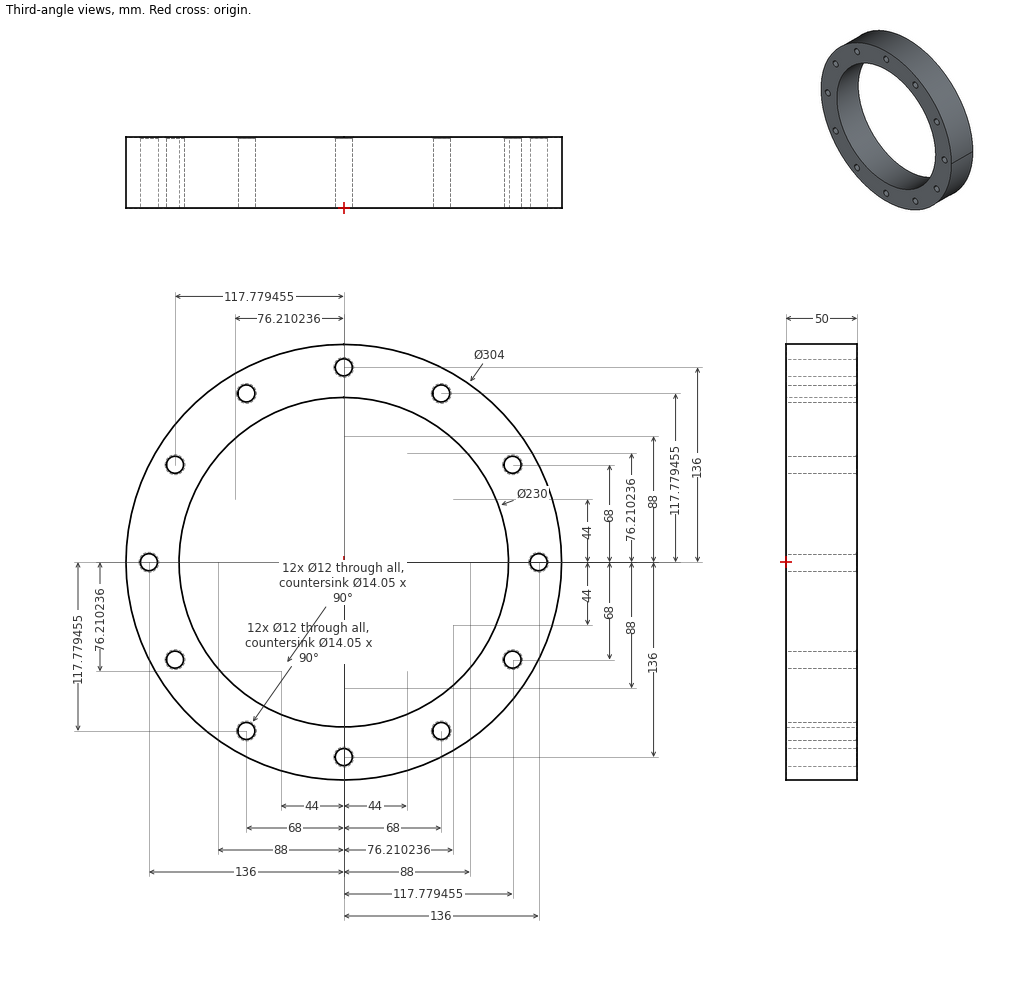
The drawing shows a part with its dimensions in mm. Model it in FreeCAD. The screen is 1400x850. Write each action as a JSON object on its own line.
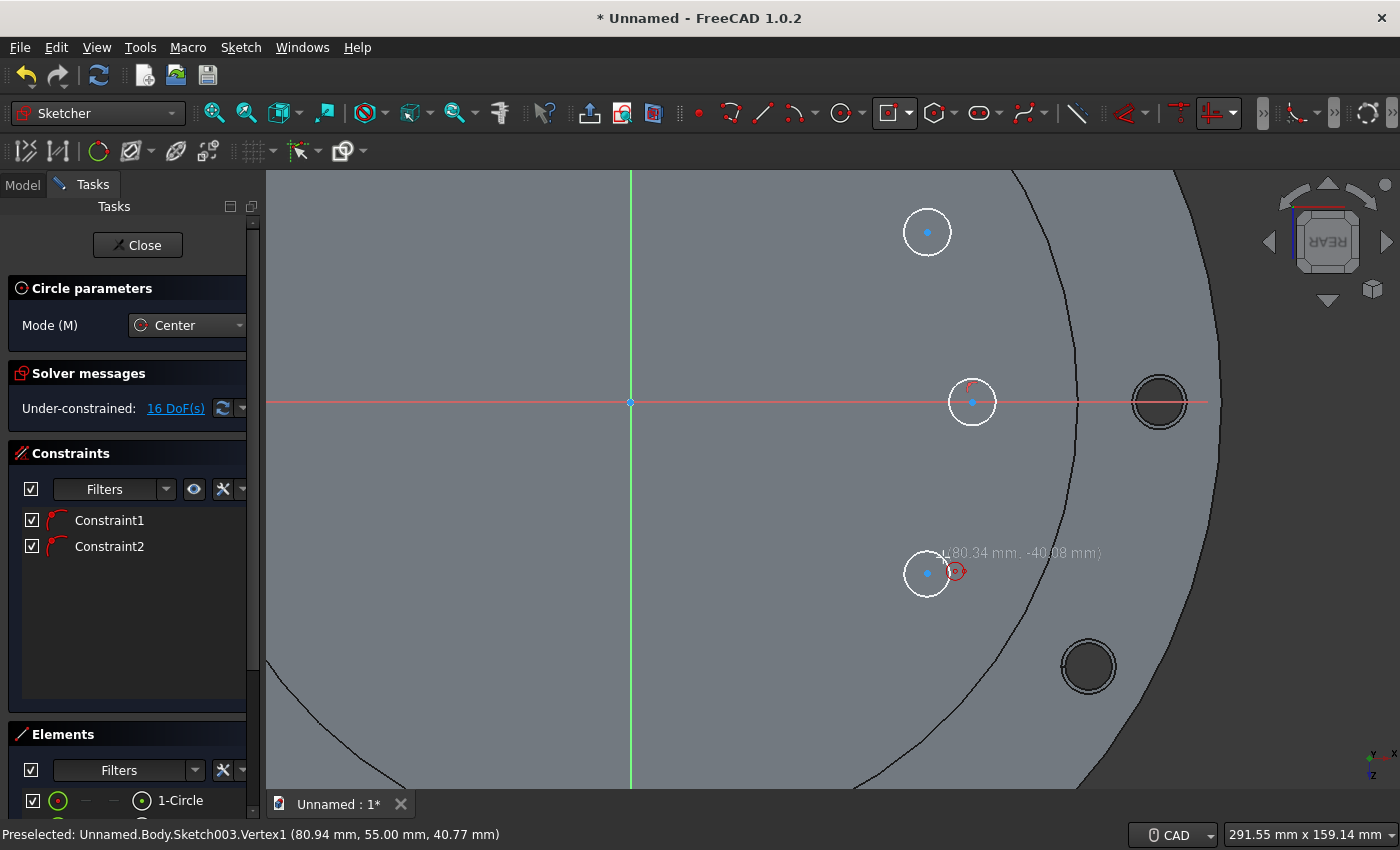
{"action": "left_click", "coordinate": [802, 699]}
{"action": "left_click", "coordinate": [818, 682]}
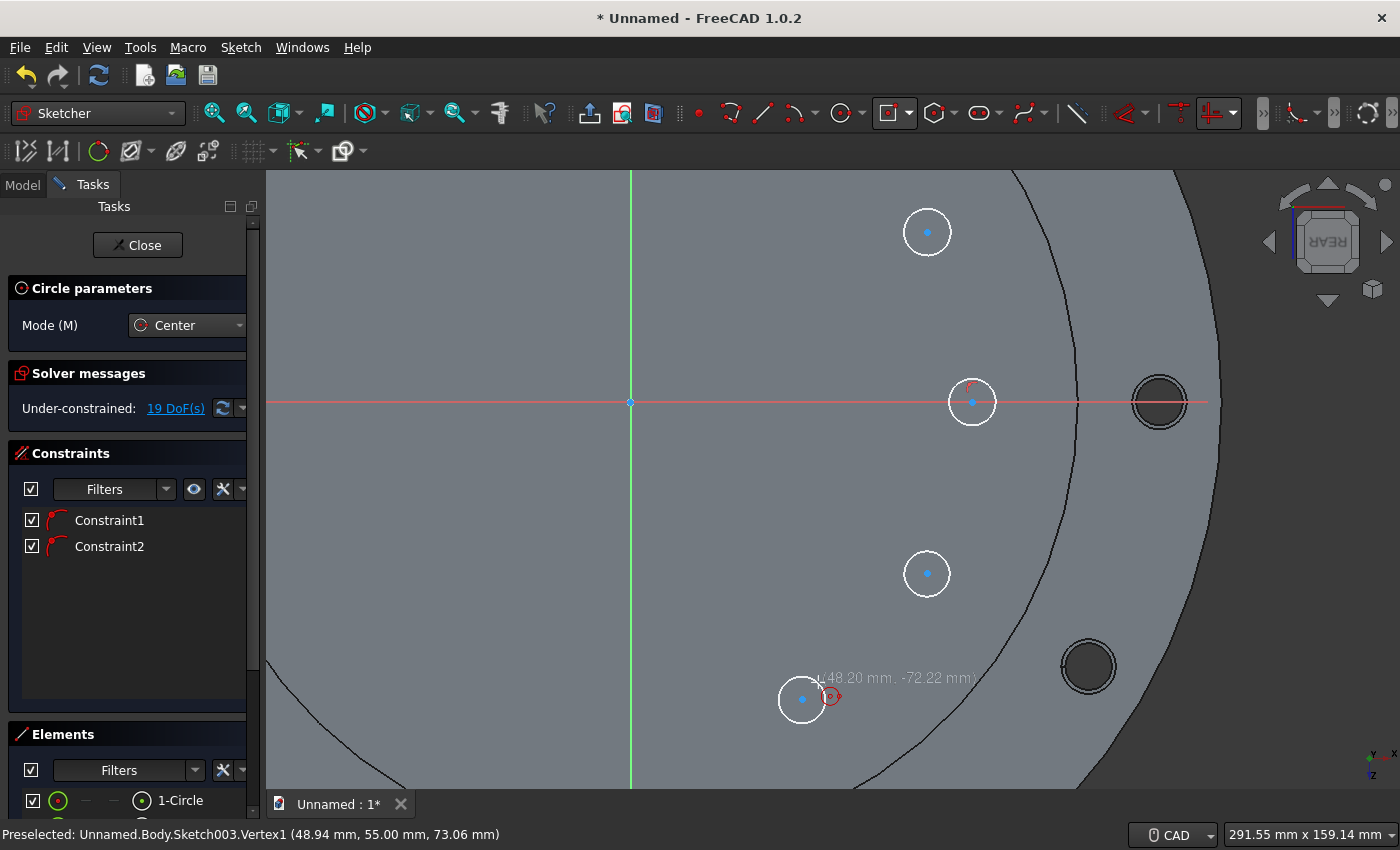
{"action": "left_click", "coordinate": [631, 744]}
{"action": "left_click", "coordinate": [647, 728]}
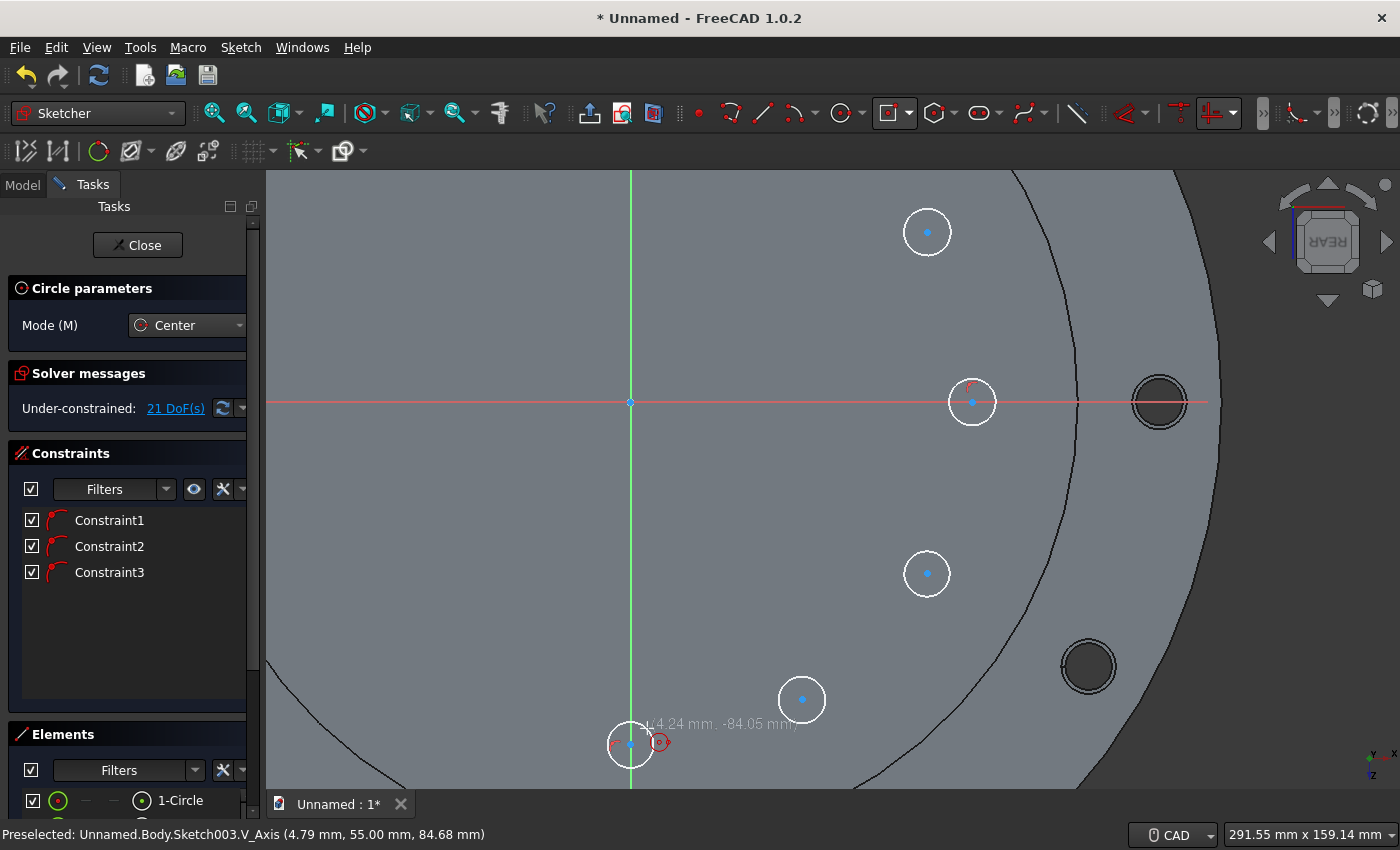
{"action": "left_click", "coordinate": [459, 699]}
{"action": "left_click", "coordinate": [476, 682]}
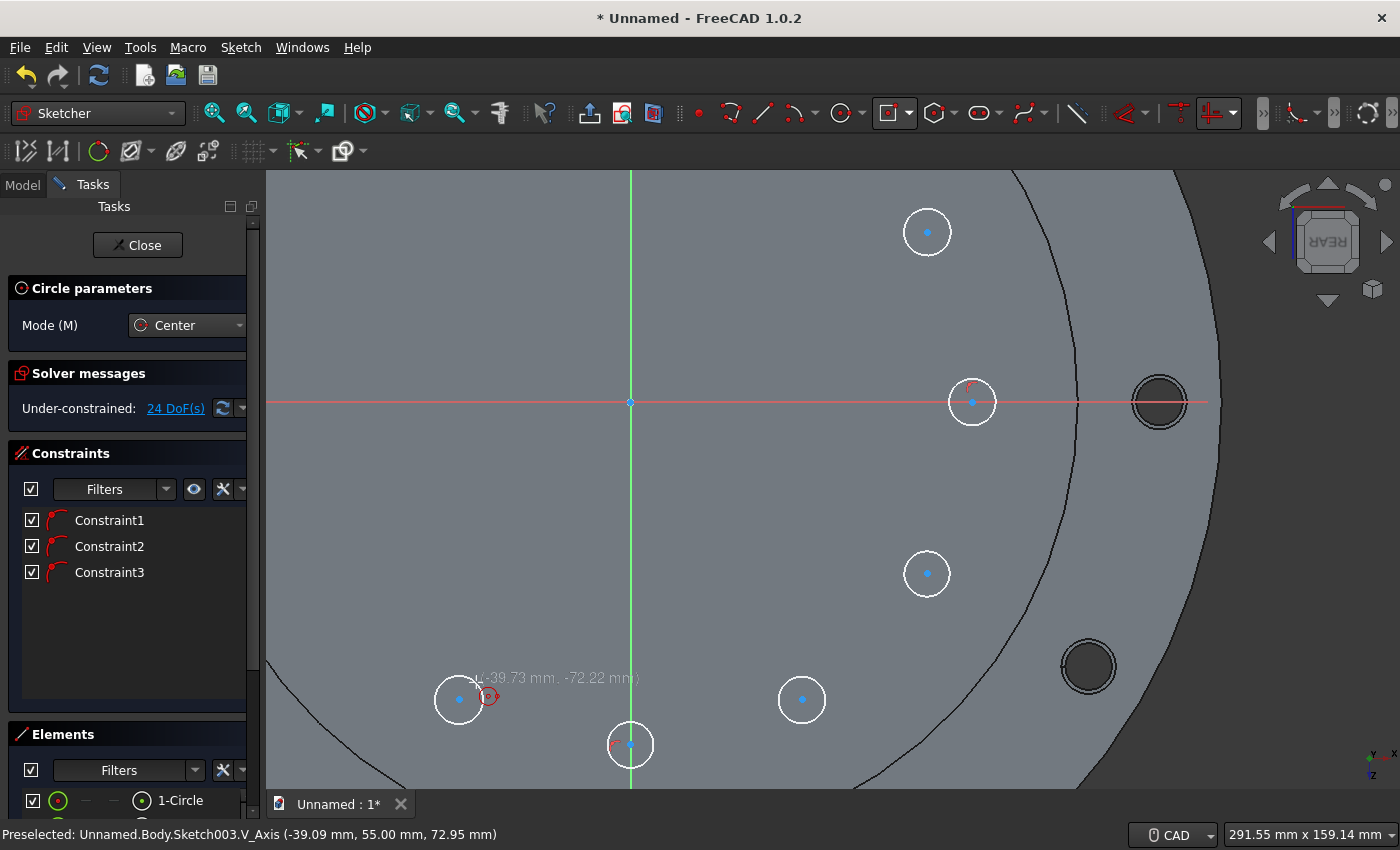
{"action": "left_click", "coordinate": [334, 573]}
{"action": "left_click", "coordinate": [351, 557]}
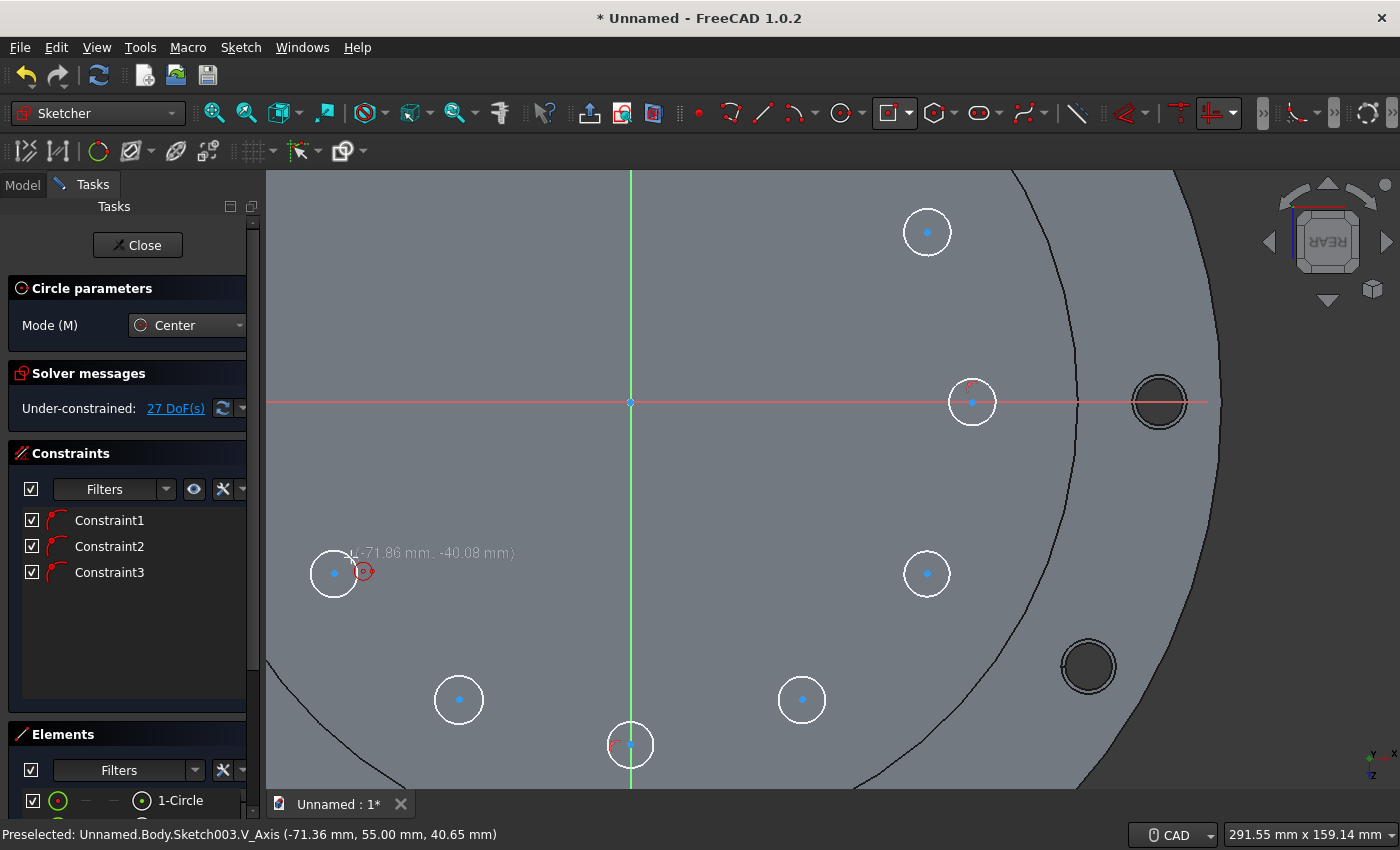
{"action": "scroll", "coordinate": [927, 574], "scroll_direction": "down", "scroll_amount": 3}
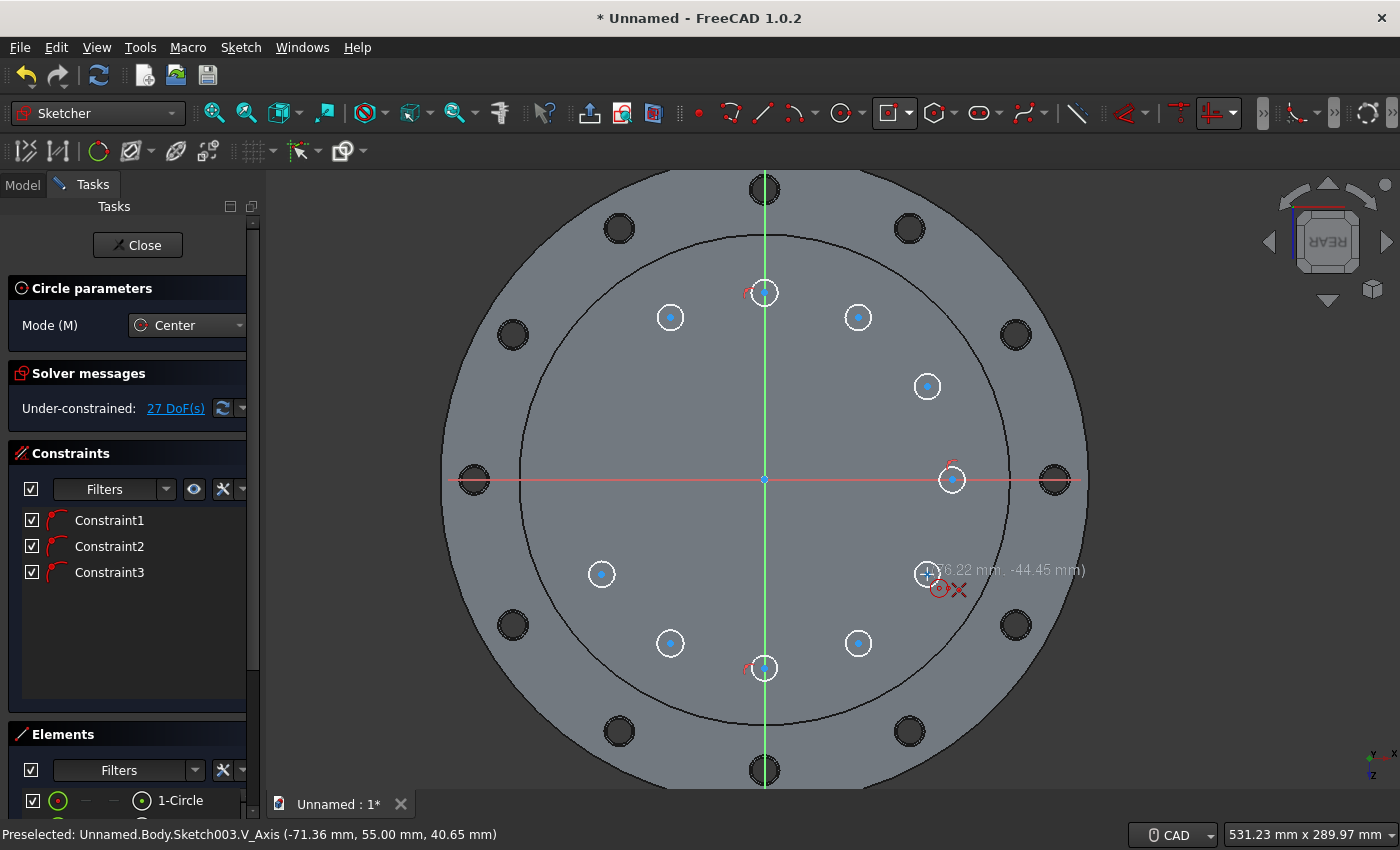
{"action": "scroll", "coordinate": [577, 480], "scroll_direction": "up", "scroll_amount": 3}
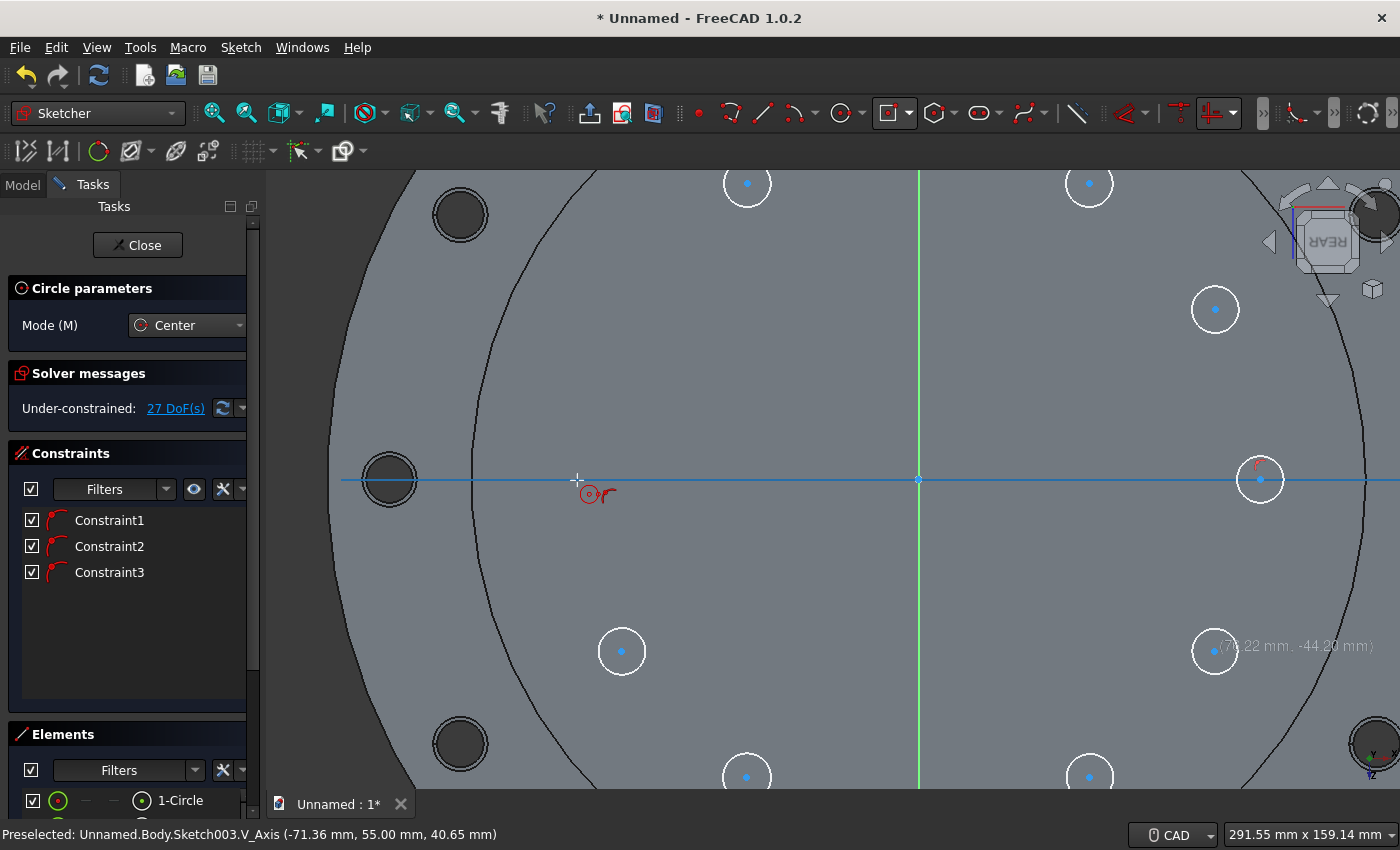
{"action": "left_click", "coordinate": [576, 479]}
{"action": "left_click", "coordinate": [593, 463]}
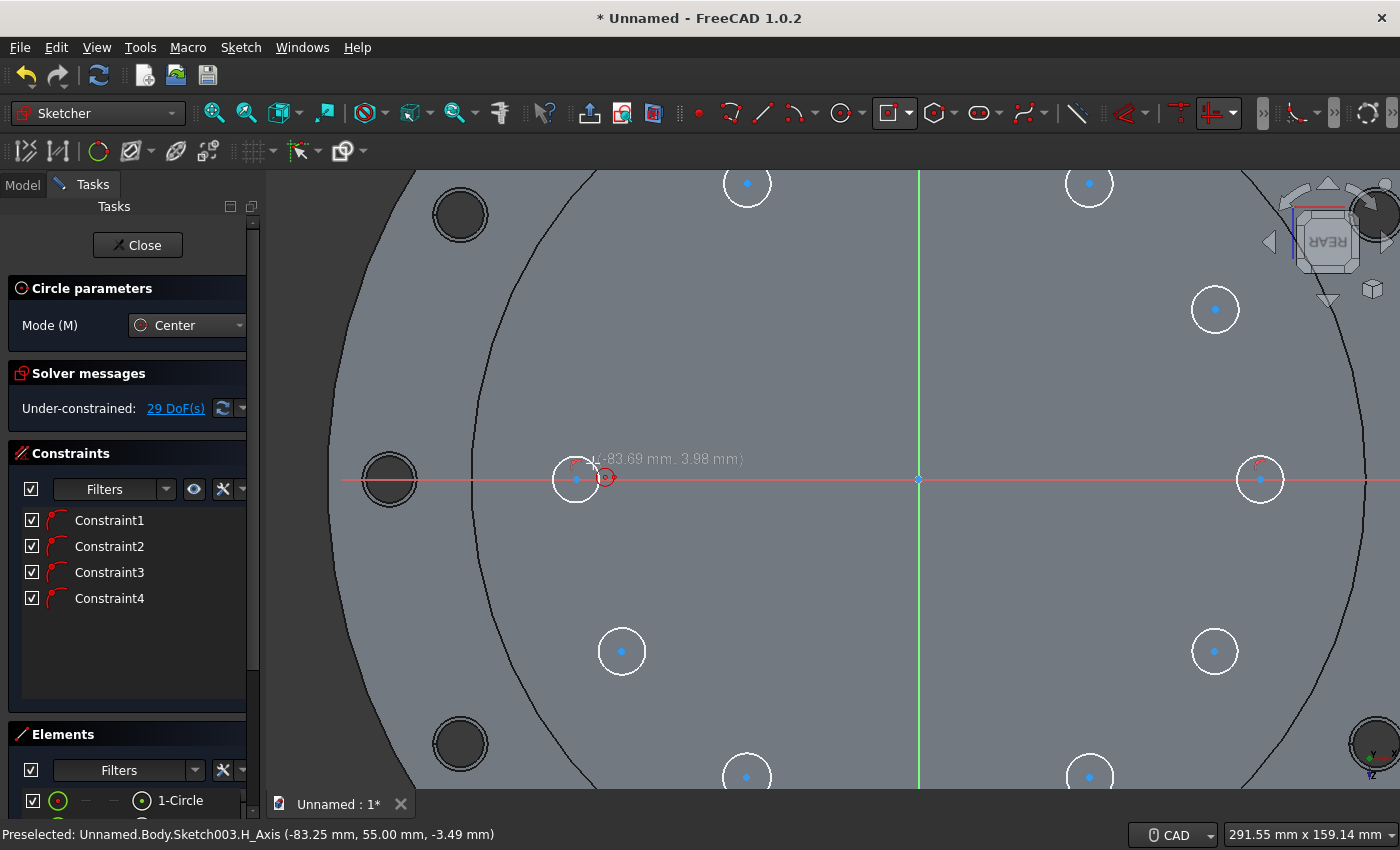
{"action": "left_click", "coordinate": [622, 308]}
{"action": "left_click", "coordinate": [639, 292]}
{"action": "key", "text": "Escape"}